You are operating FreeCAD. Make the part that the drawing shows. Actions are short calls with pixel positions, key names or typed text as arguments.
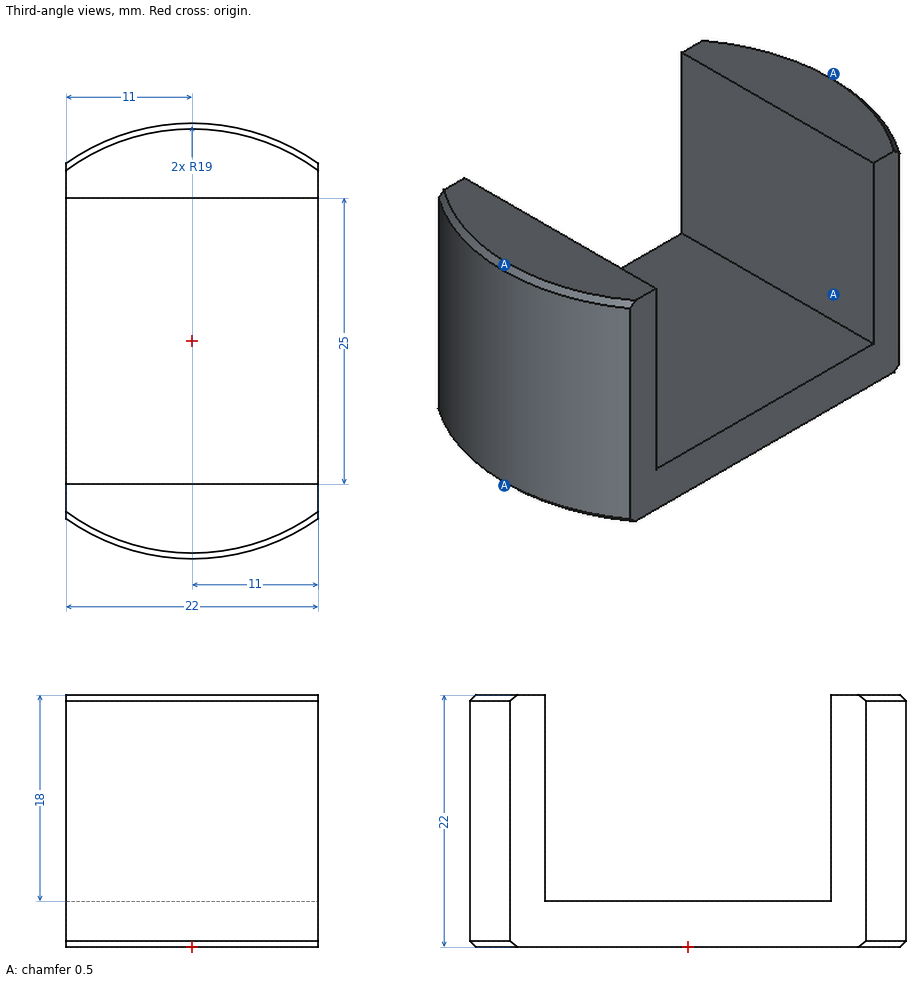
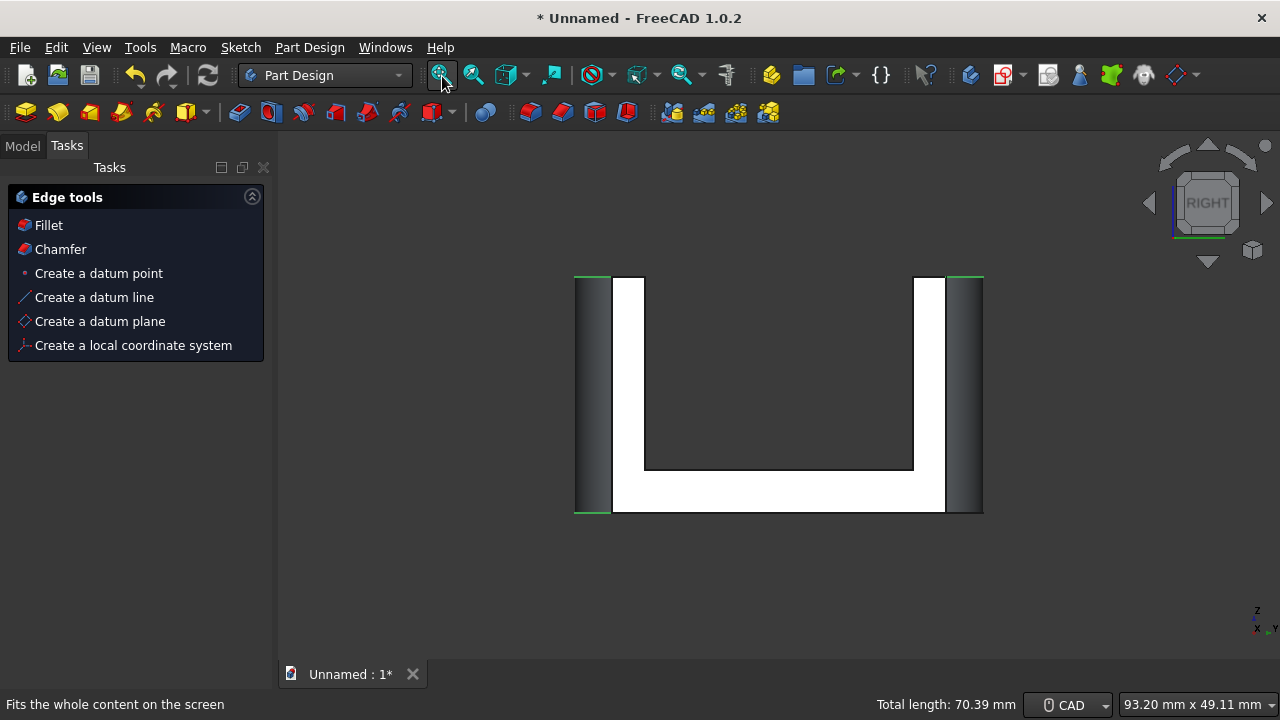
click(982, 512, ctrl)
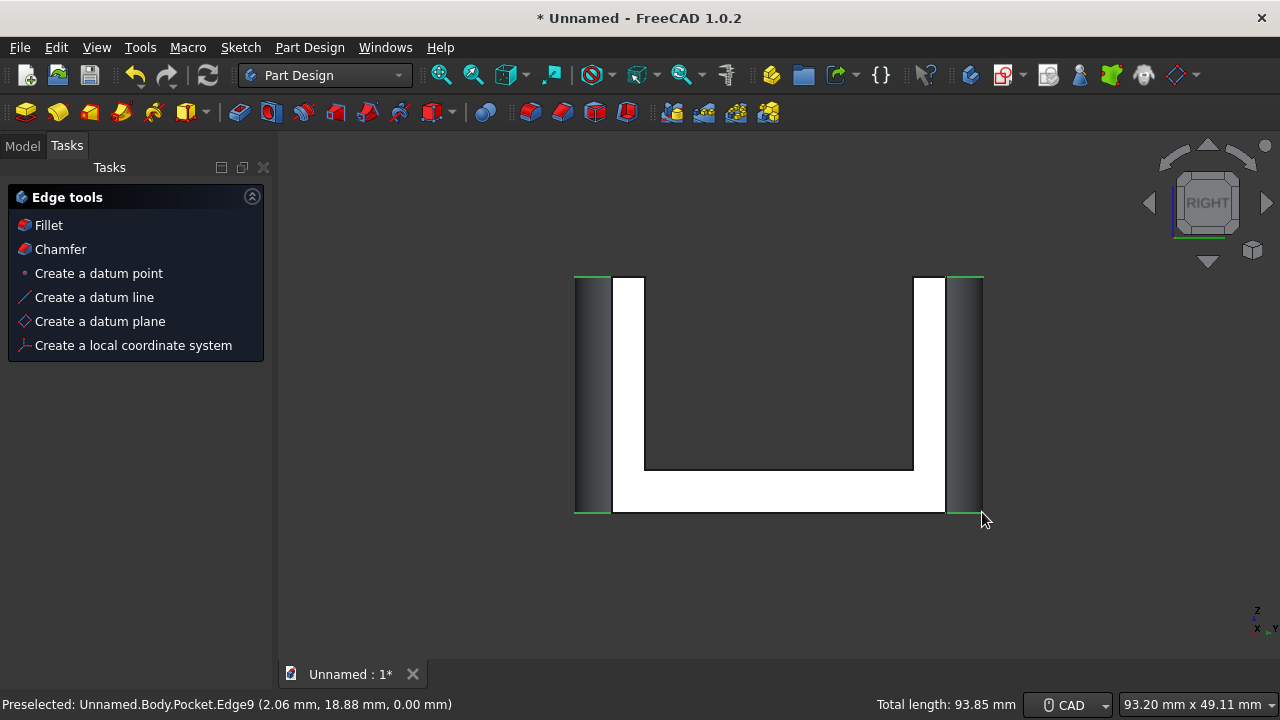
click(564, 112)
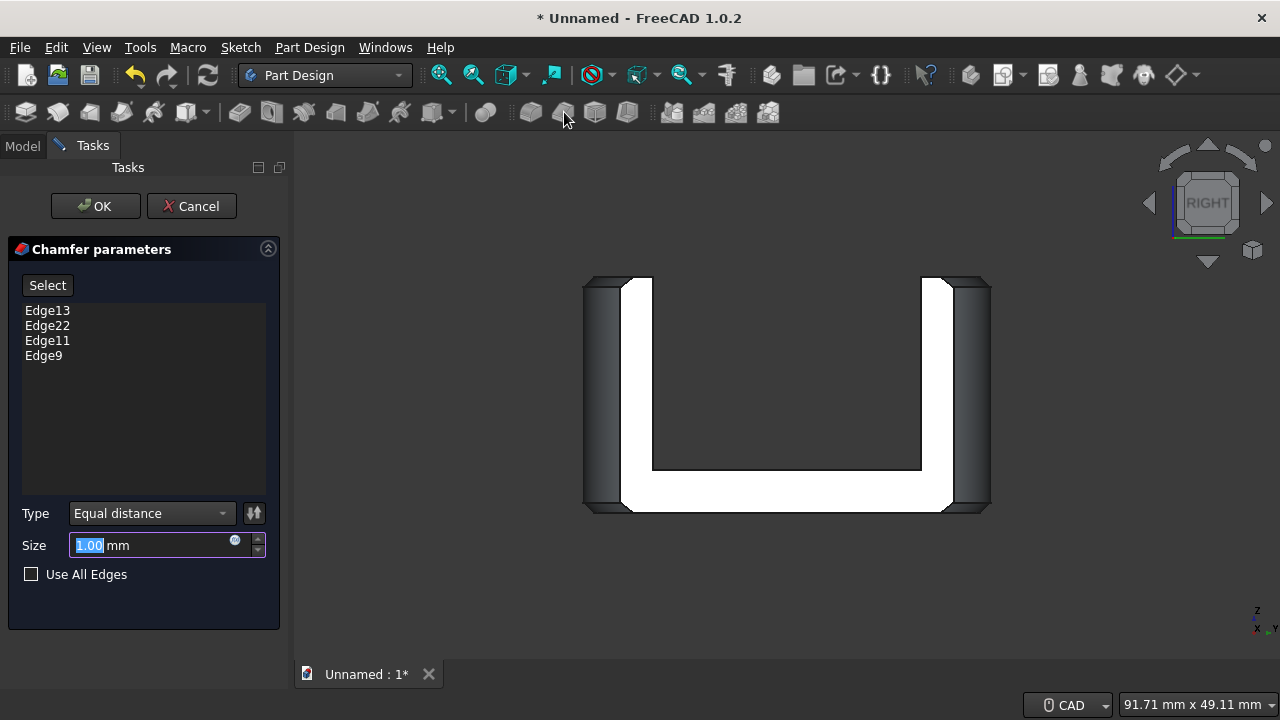
text(0.5)
key(Tab)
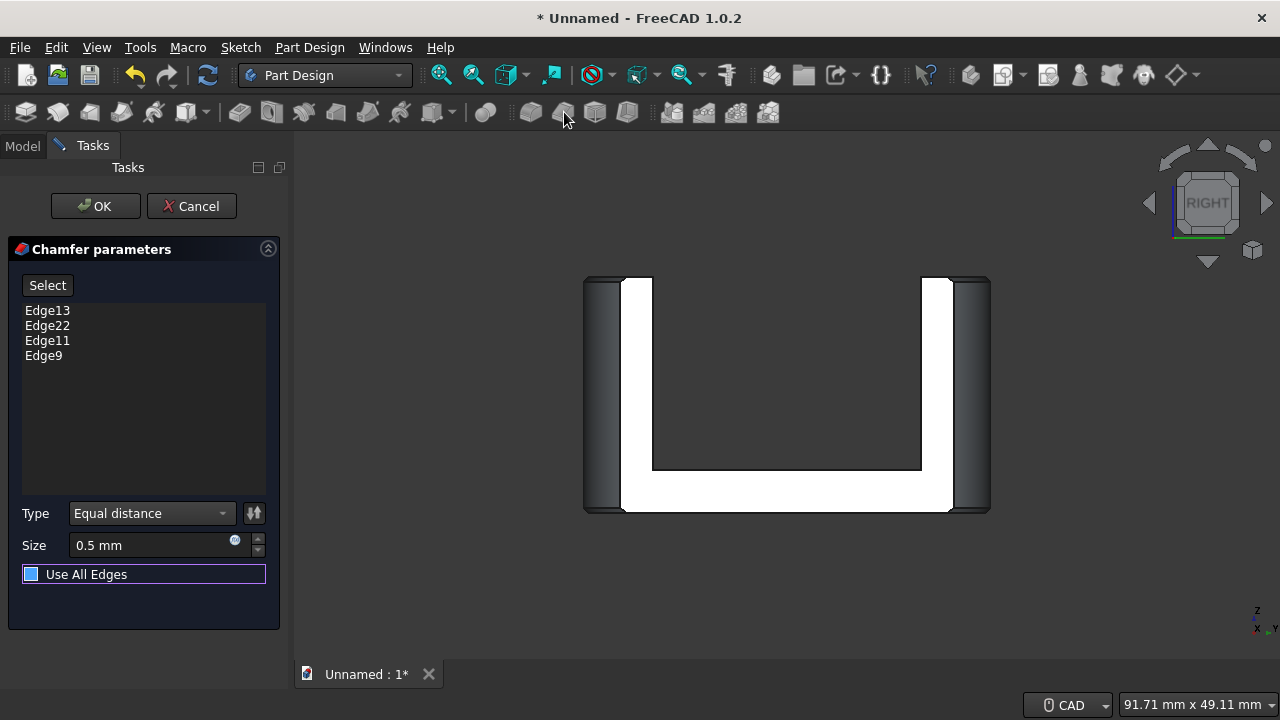
click(96, 206)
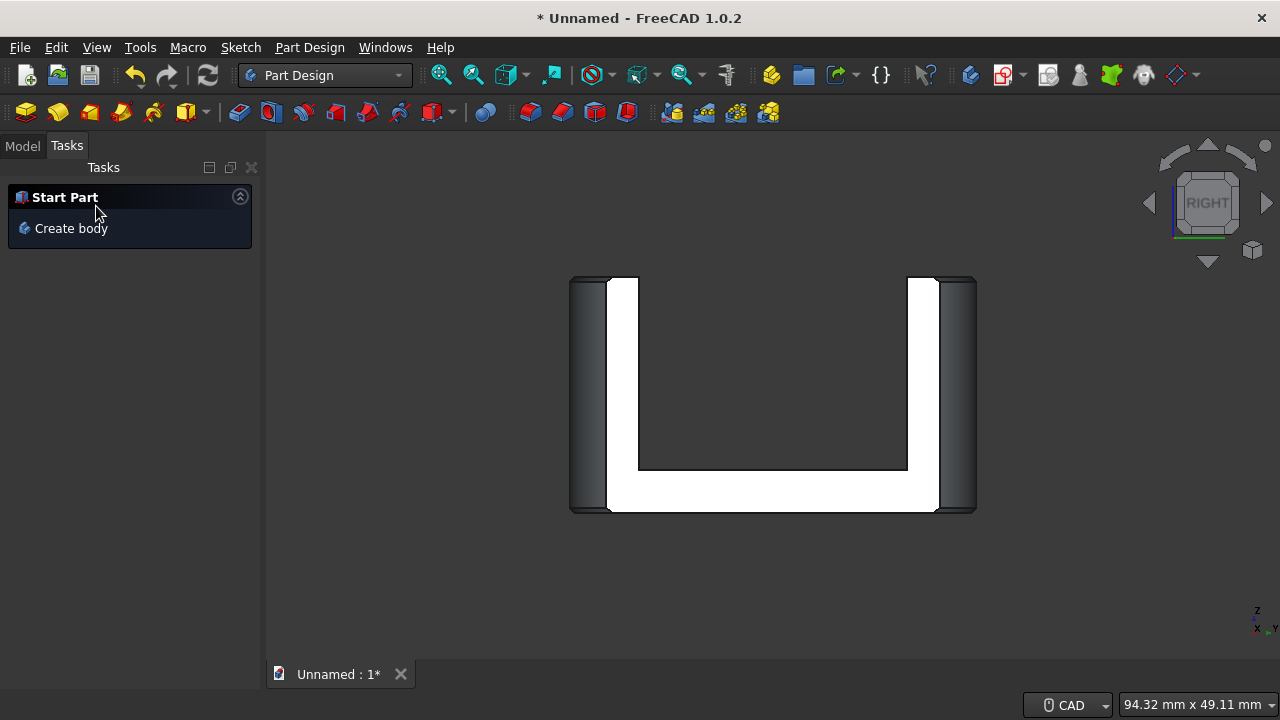
key(0)